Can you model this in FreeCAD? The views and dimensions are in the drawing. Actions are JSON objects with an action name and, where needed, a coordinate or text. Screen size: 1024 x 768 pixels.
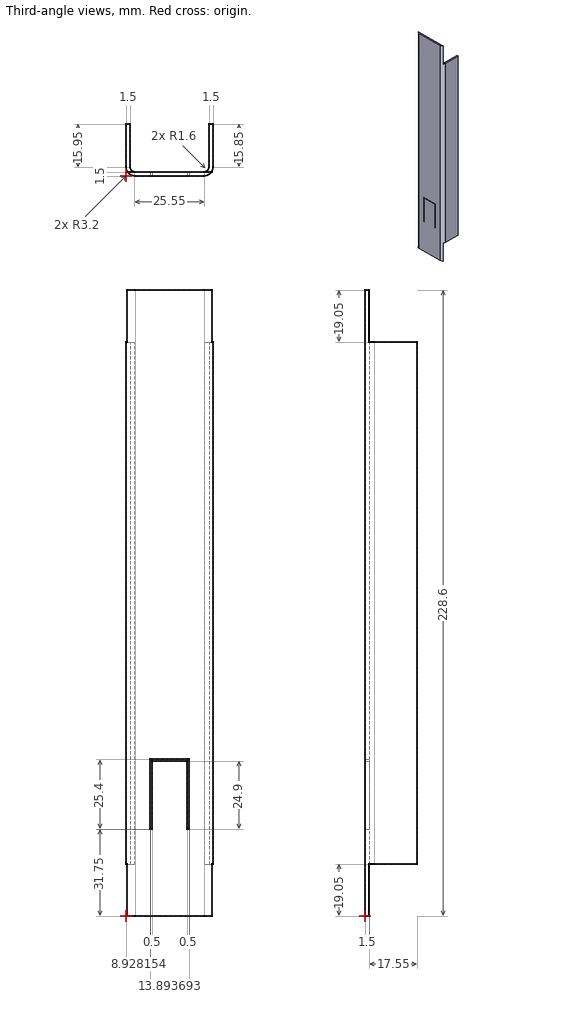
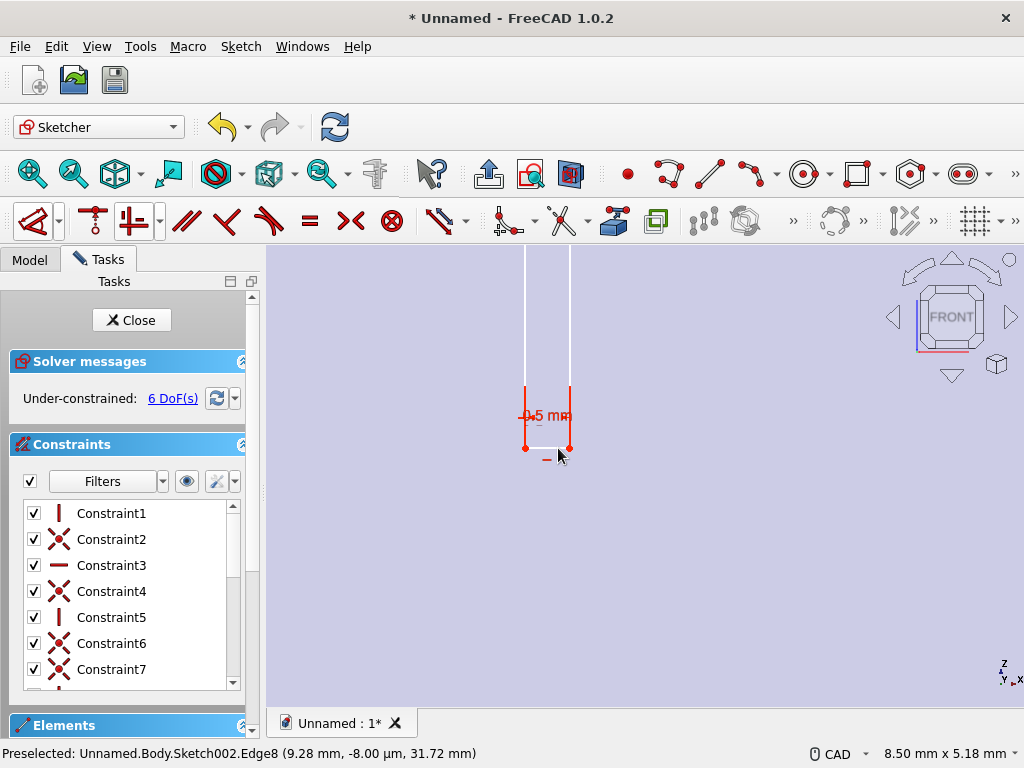
{"action": "scroll", "coordinate": [565, 460], "scroll_direction": "down", "scroll_amount": 14}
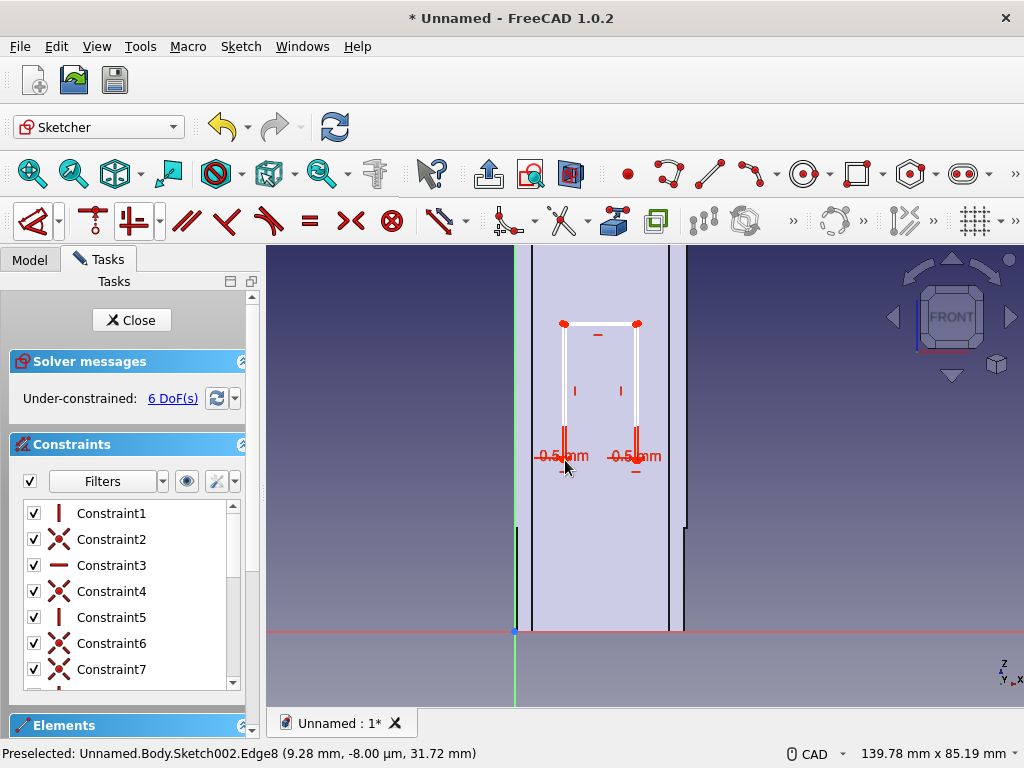
{"action": "scroll", "coordinate": [563, 419], "scroll_direction": "up", "scroll_amount": 9}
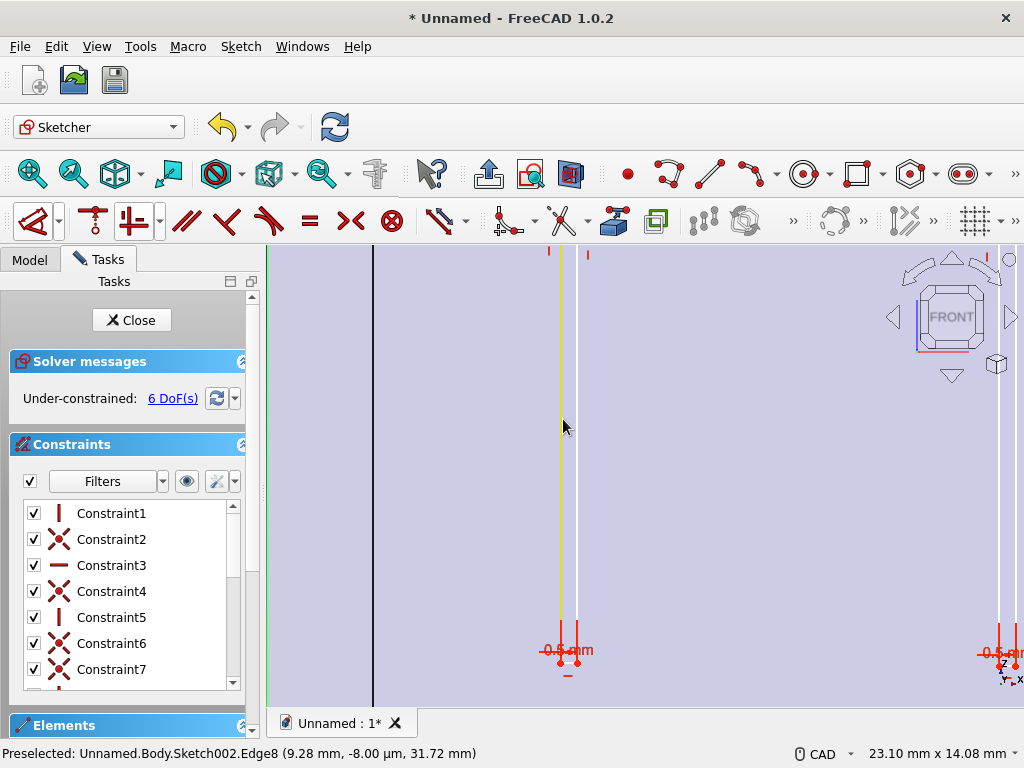
{"action": "left_click", "coordinate": [561, 416]}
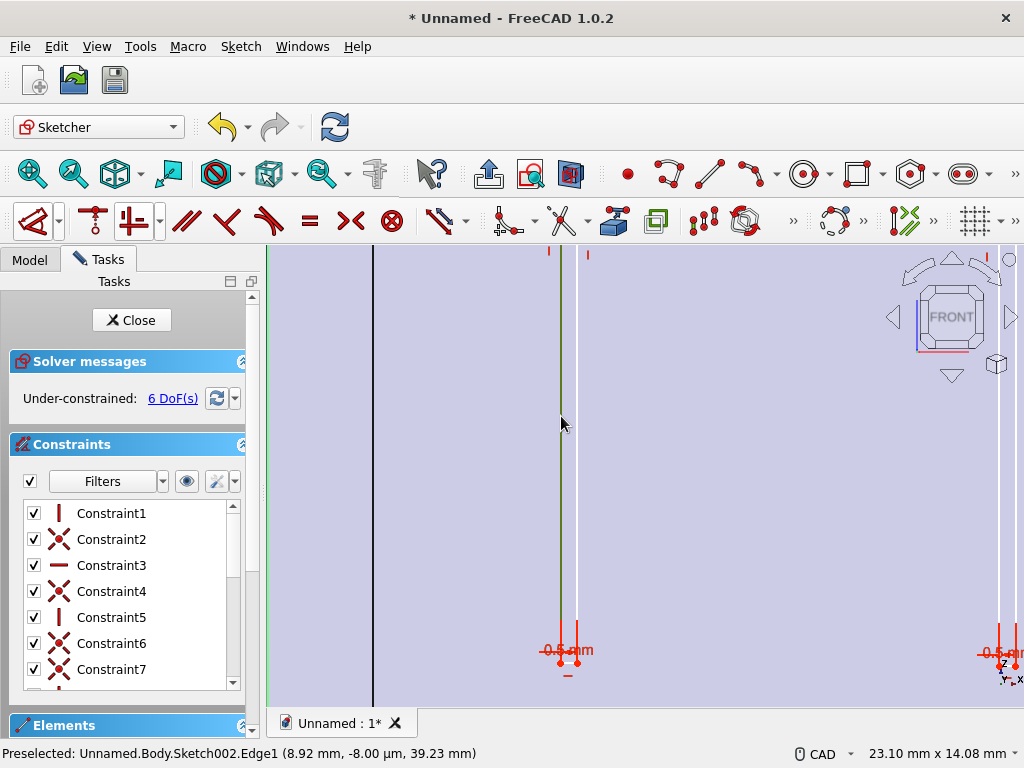
{"action": "left_click", "coordinate": [58, 222]}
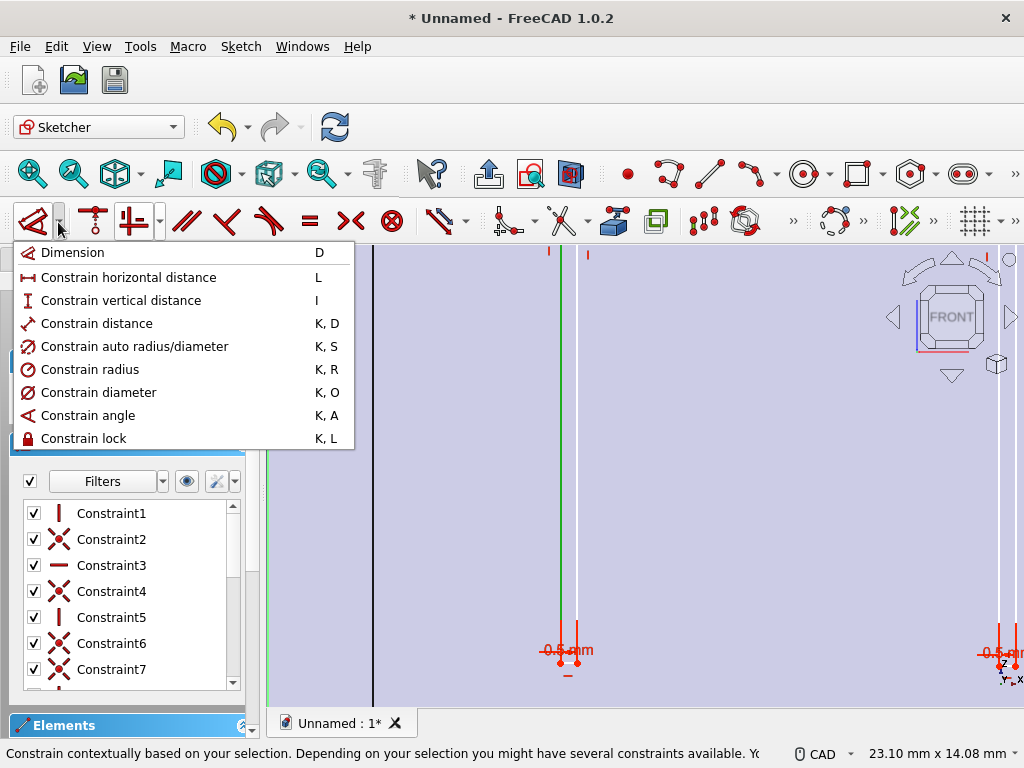
{"action": "left_click", "coordinate": [184, 300]}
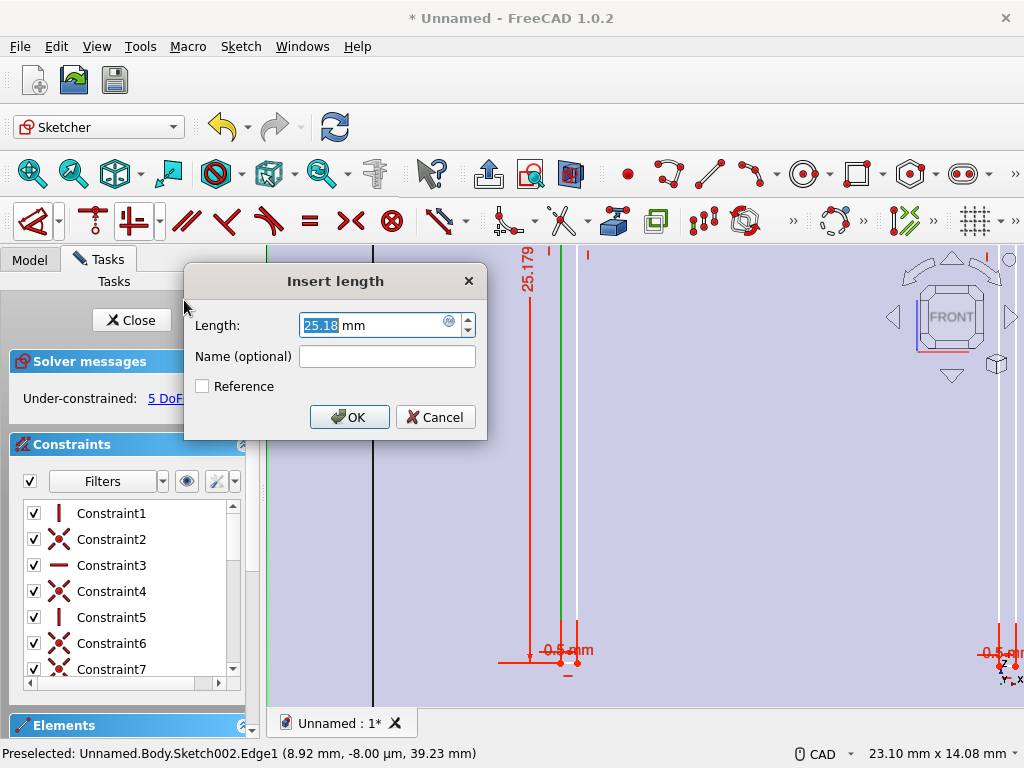
{"action": "type", "text": "25.4"}
{"action": "key", "text": "Return"}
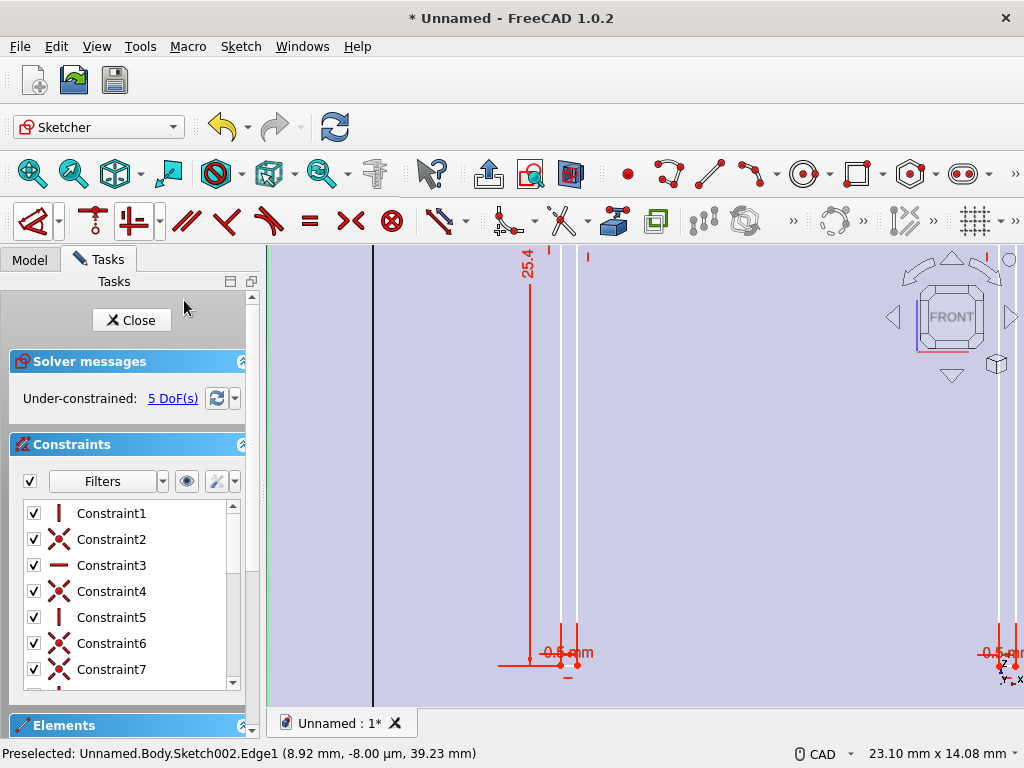
{"action": "scroll", "coordinate": [563, 418], "scroll_direction": "down", "scroll_amount": 9}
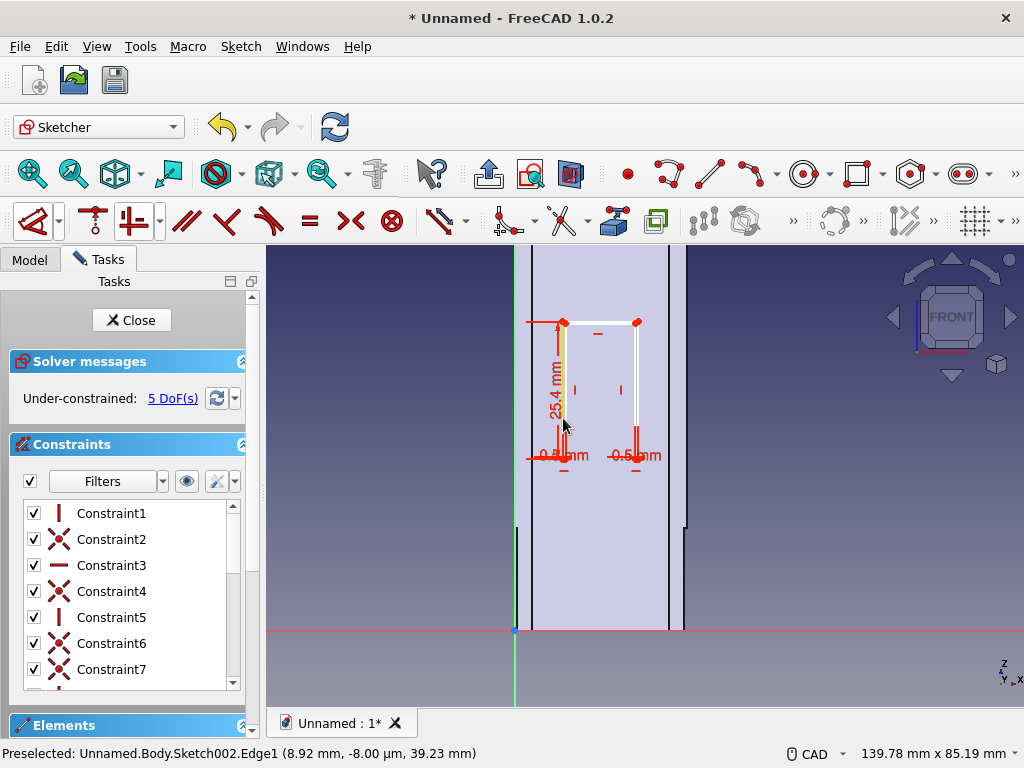
{"action": "scroll", "coordinate": [638, 363], "scroll_direction": "up", "scroll_amount": 9}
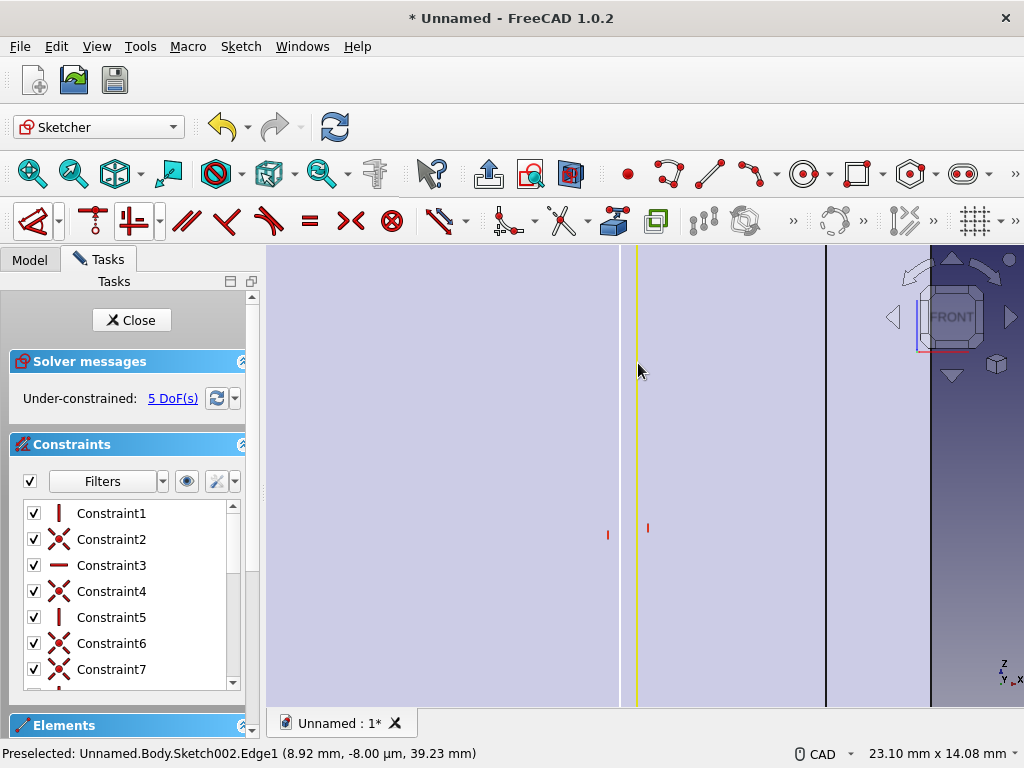
{"action": "left_click", "coordinate": [637, 361]}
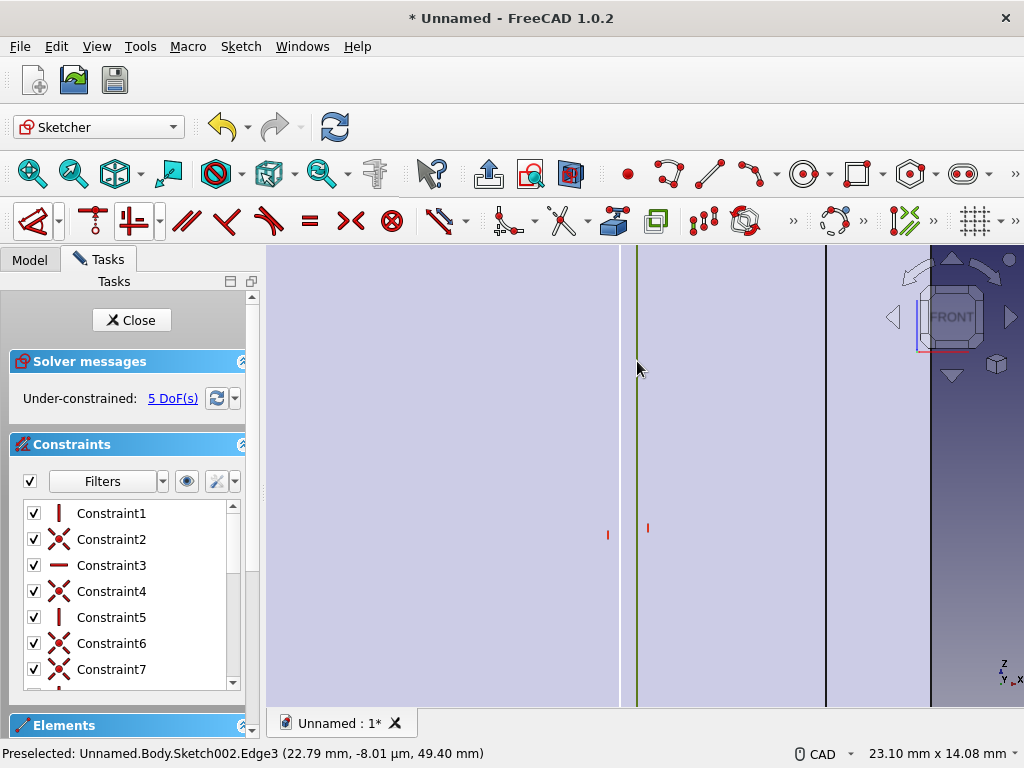
{"action": "left_click", "coordinate": [58, 222]}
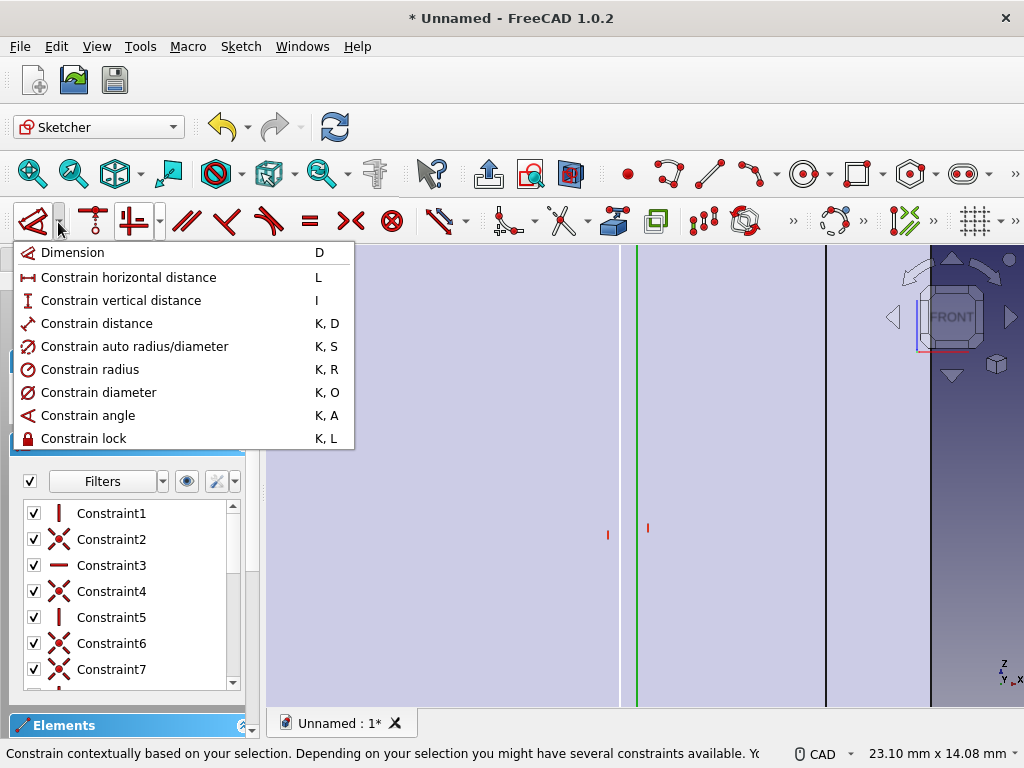
{"action": "left_click", "coordinate": [184, 300]}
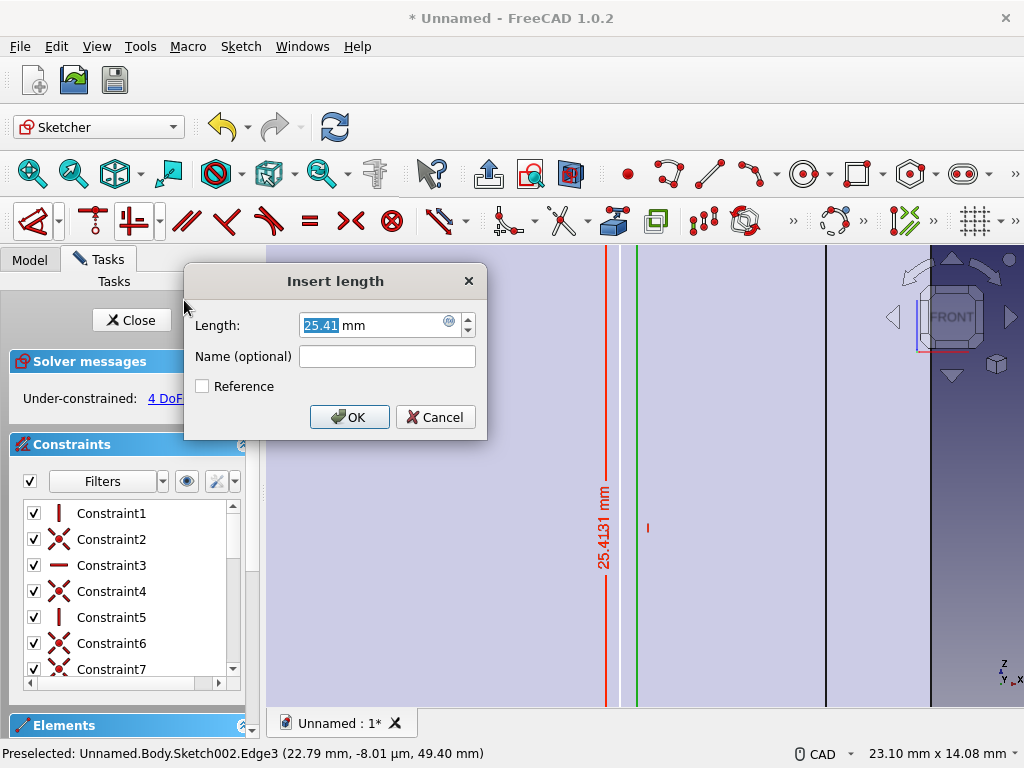
{"action": "type", "text": "25.4"}
{"action": "key", "text": "Return"}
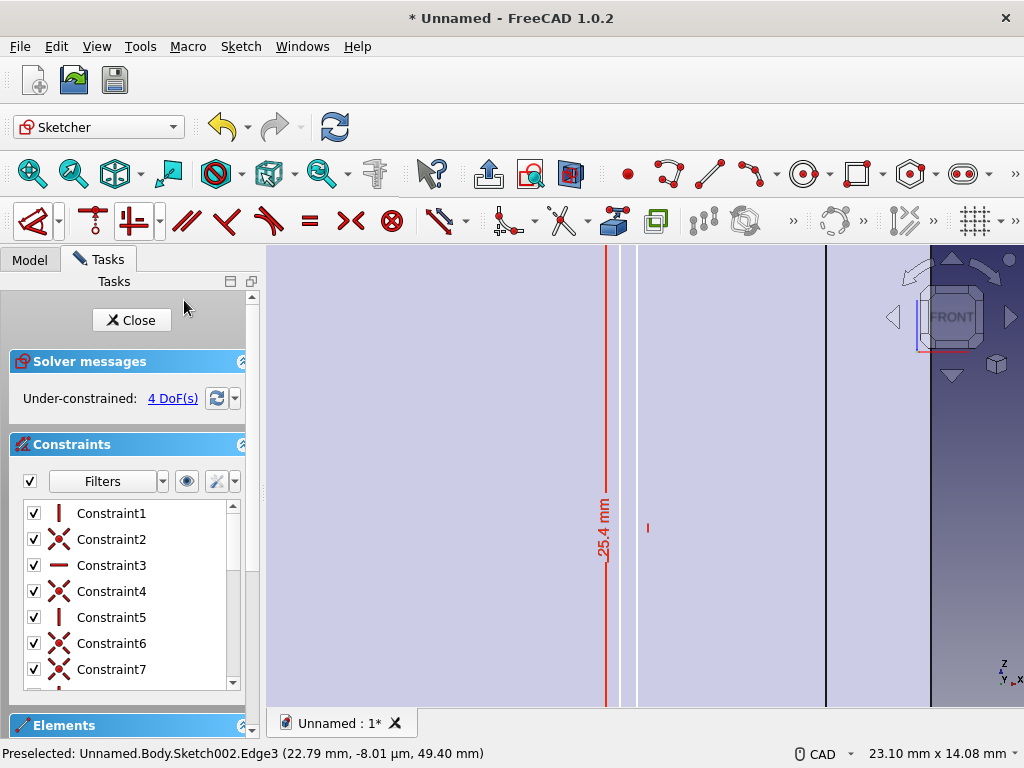
{"action": "left_click", "coordinate": [620, 370]}